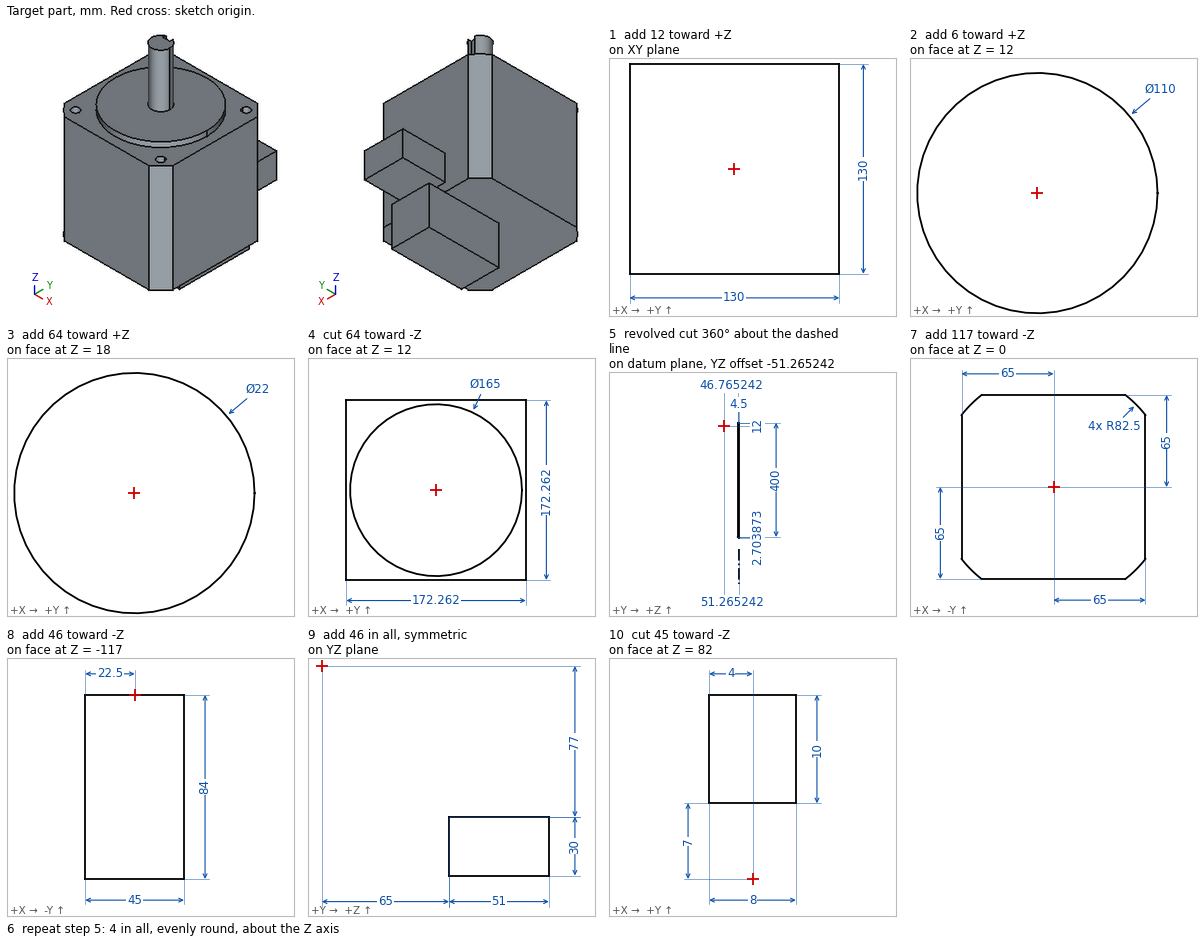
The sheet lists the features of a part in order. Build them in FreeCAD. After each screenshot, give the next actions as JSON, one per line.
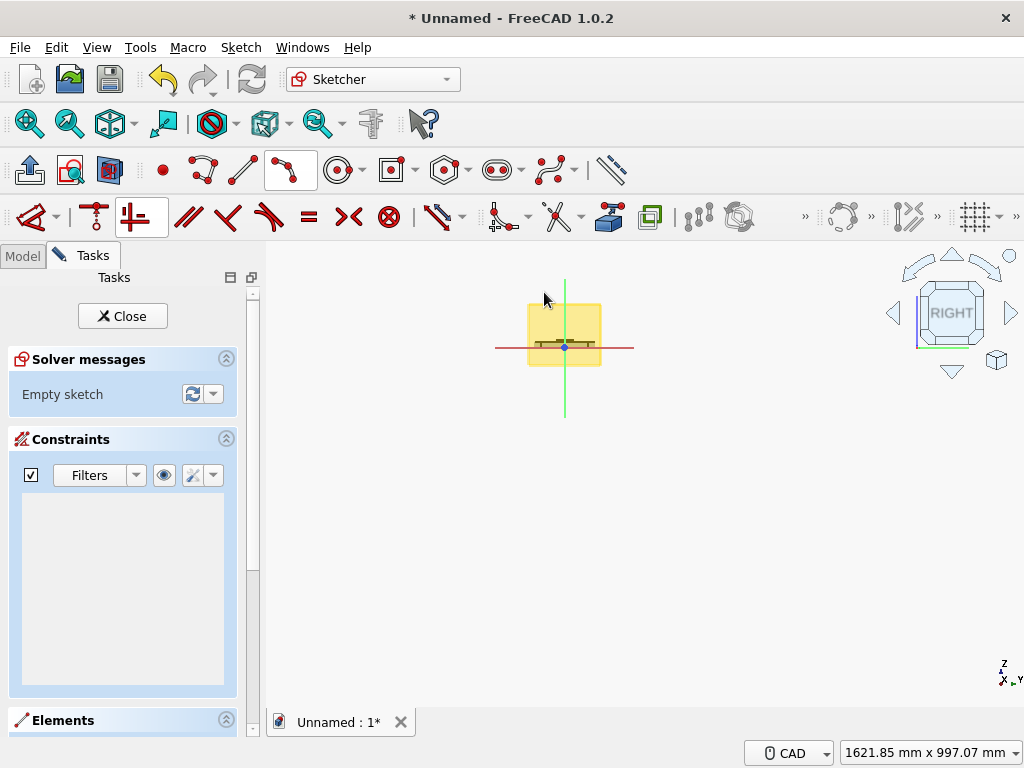
{"action": "left_click", "coordinate": [204, 170]}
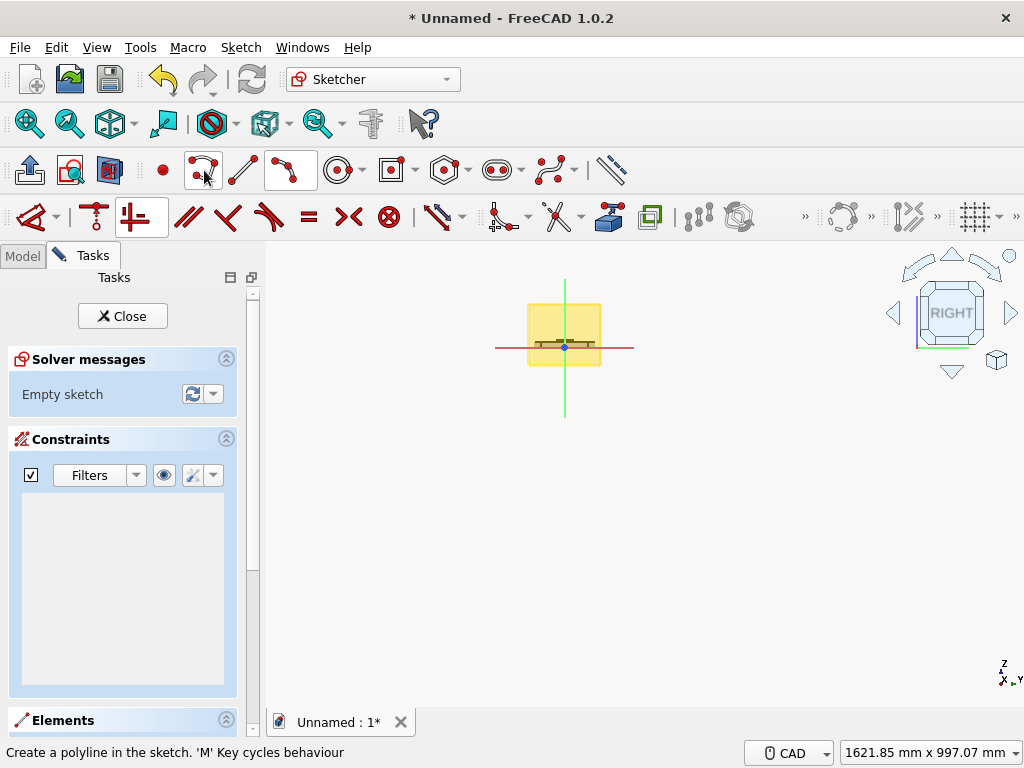
{"action": "scroll", "coordinate": [587, 342], "scroll_direction": "up", "scroll_amount": 6}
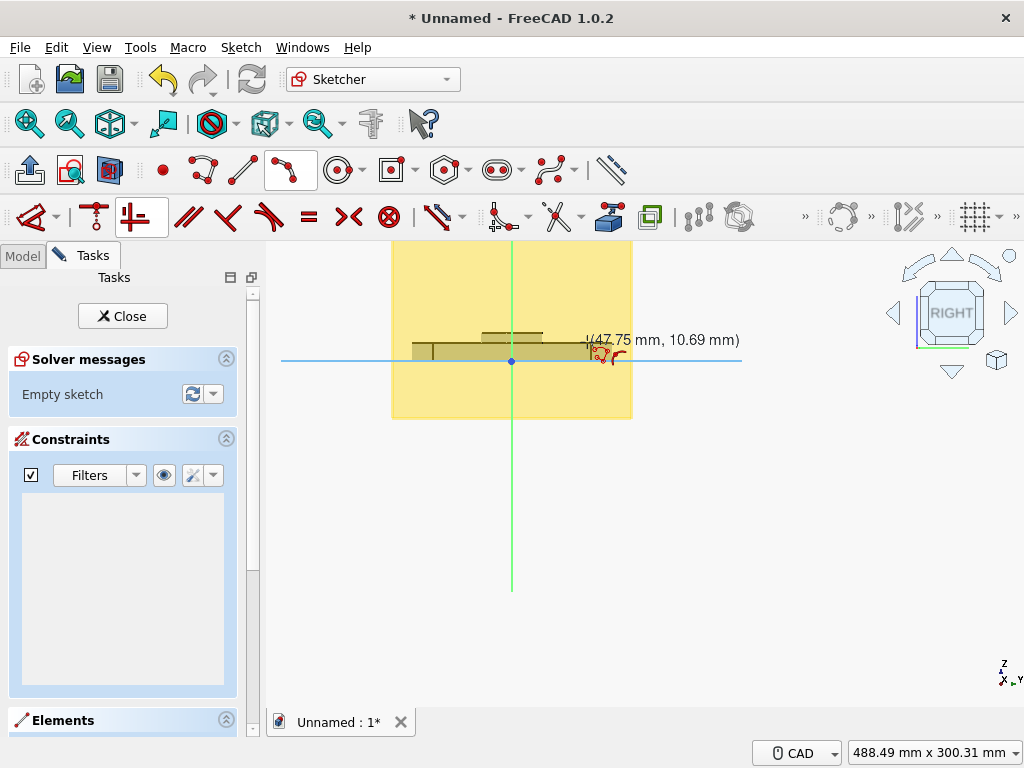
{"action": "left_click", "coordinate": [584, 343]}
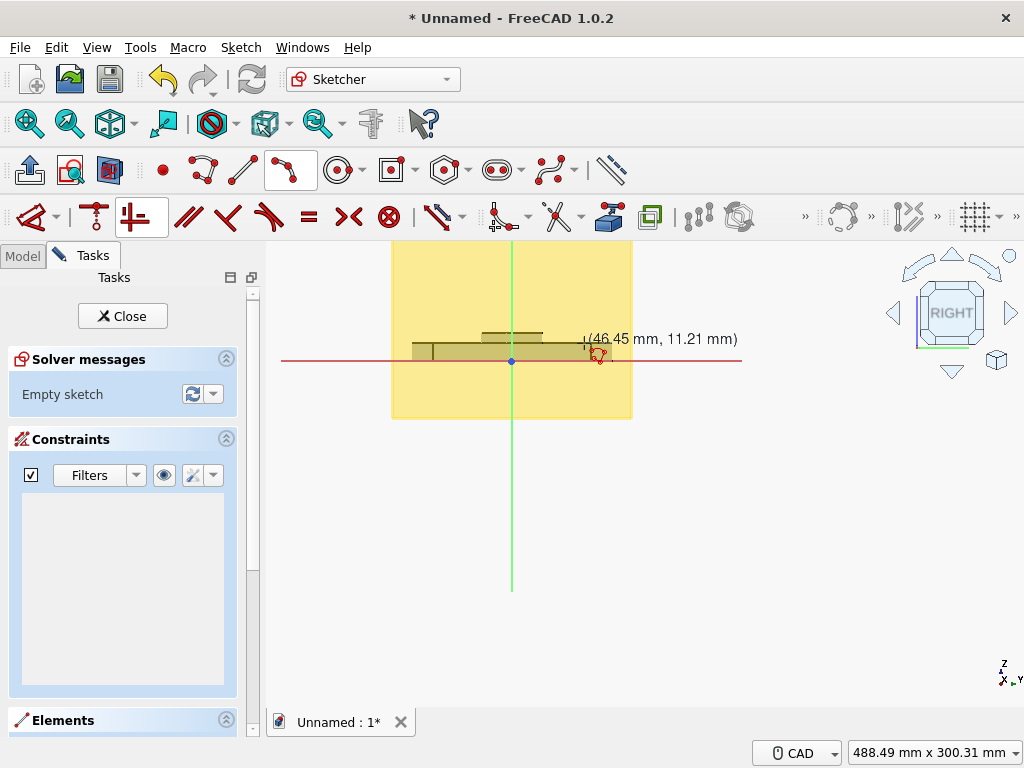
{"action": "scroll", "coordinate": [587, 342], "scroll_direction": "down", "scroll_amount": 6}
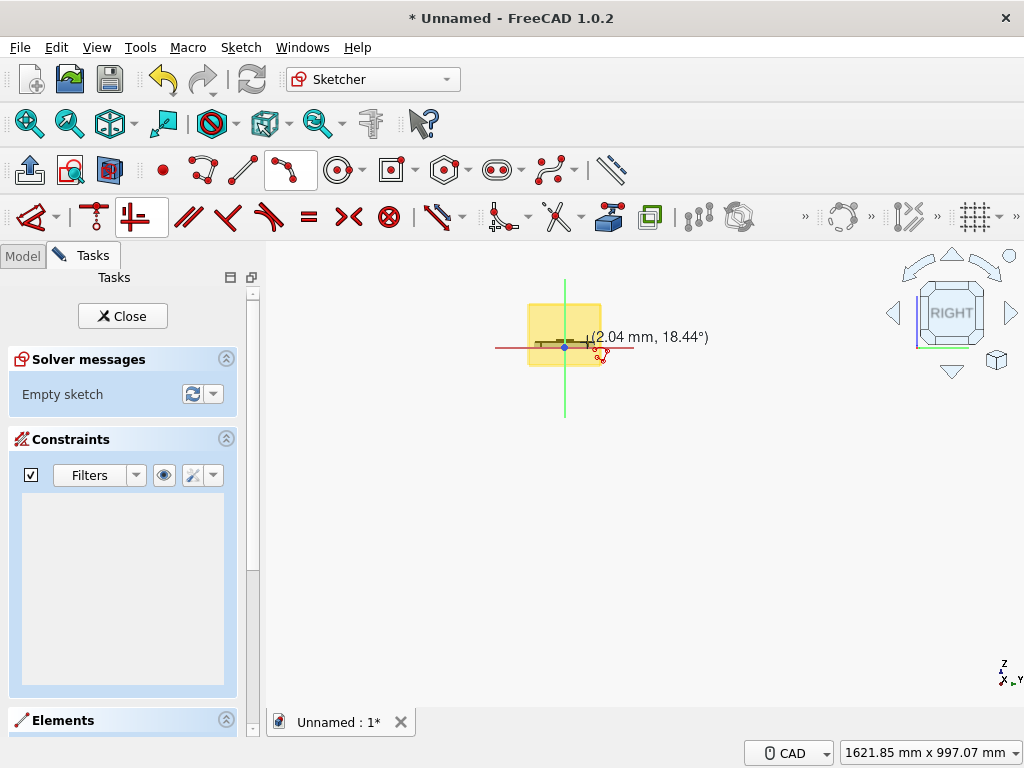
{"action": "left_click", "coordinate": [586, 529]}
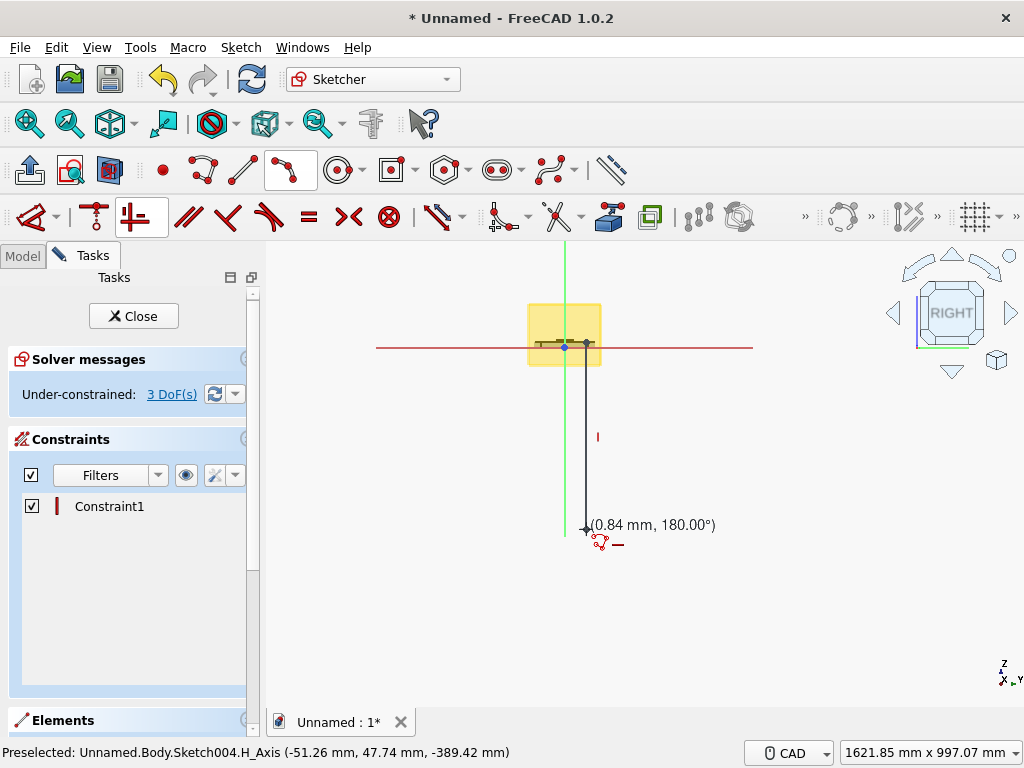
{"action": "scroll", "coordinate": [589, 531], "scroll_direction": "up", "scroll_amount": 10}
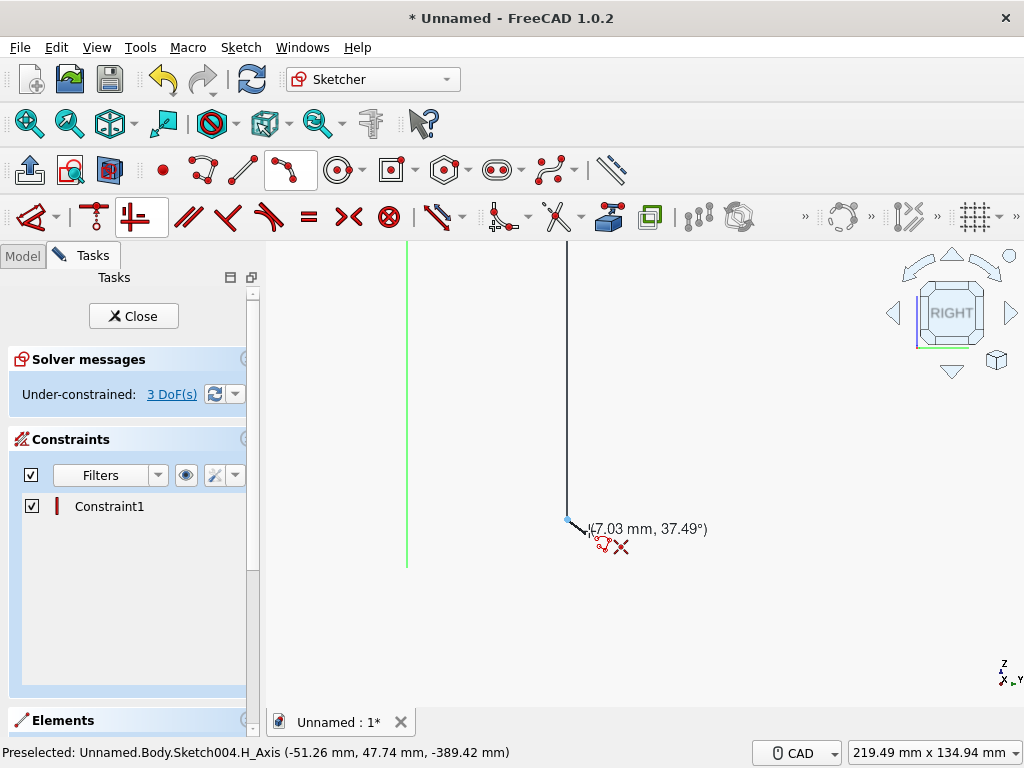
{"action": "left_click", "coordinate": [584, 524]}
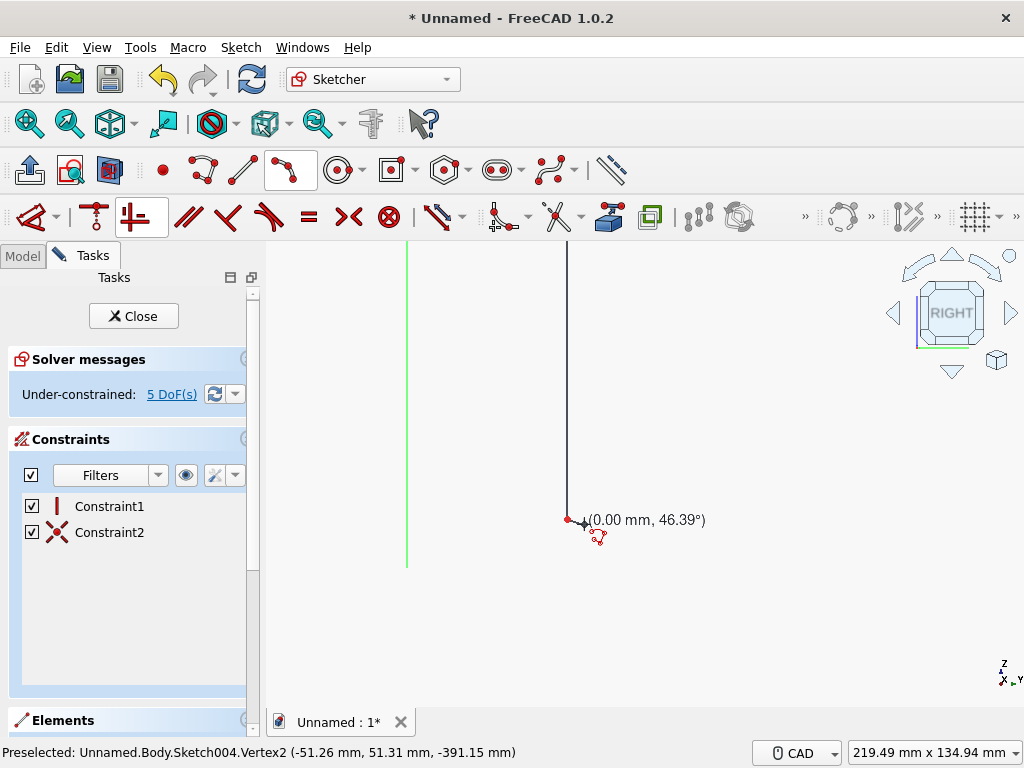
{"action": "scroll", "coordinate": [589, 531], "scroll_direction": "down", "scroll_amount": 10}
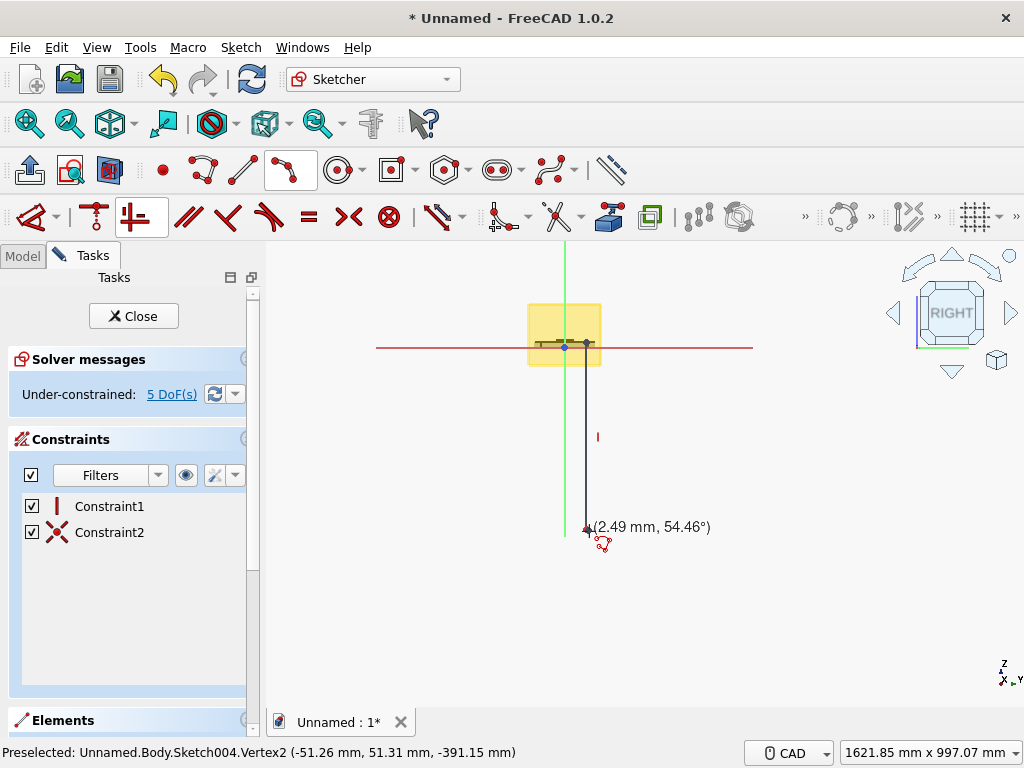
{"action": "scroll", "coordinate": [589, 342], "scroll_direction": "up", "scroll_amount": 11}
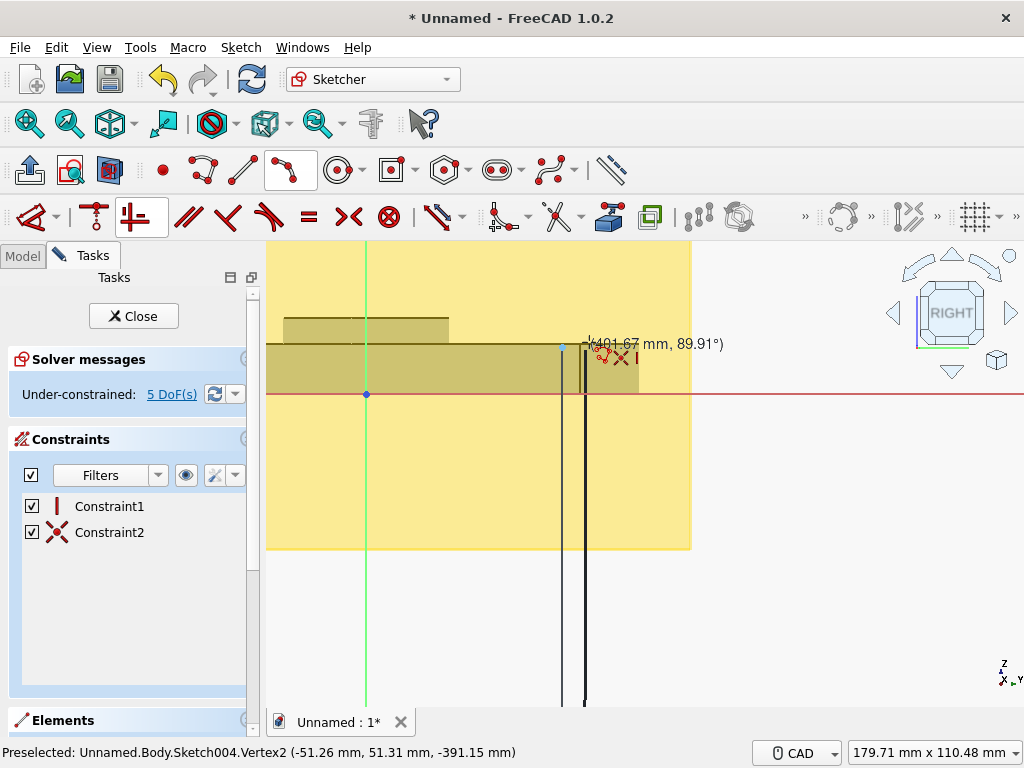
{"action": "left_click", "coordinate": [583, 344]}
{"action": "left_click", "coordinate": [562, 347]}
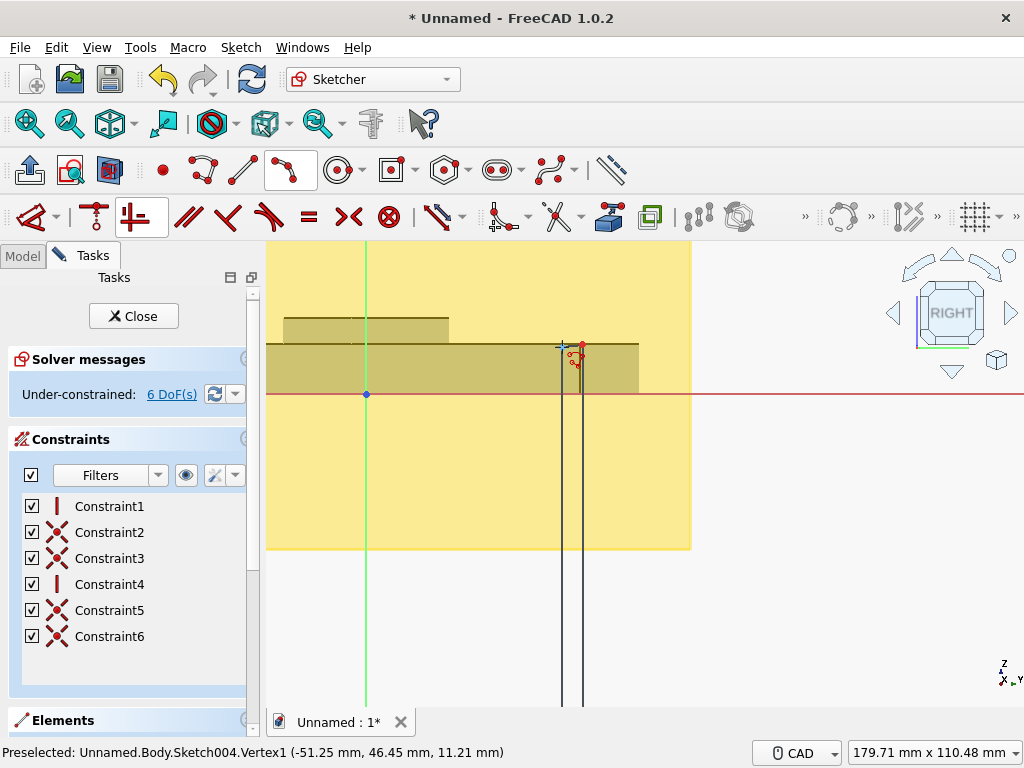
{"action": "left_click", "coordinate": [244, 170]}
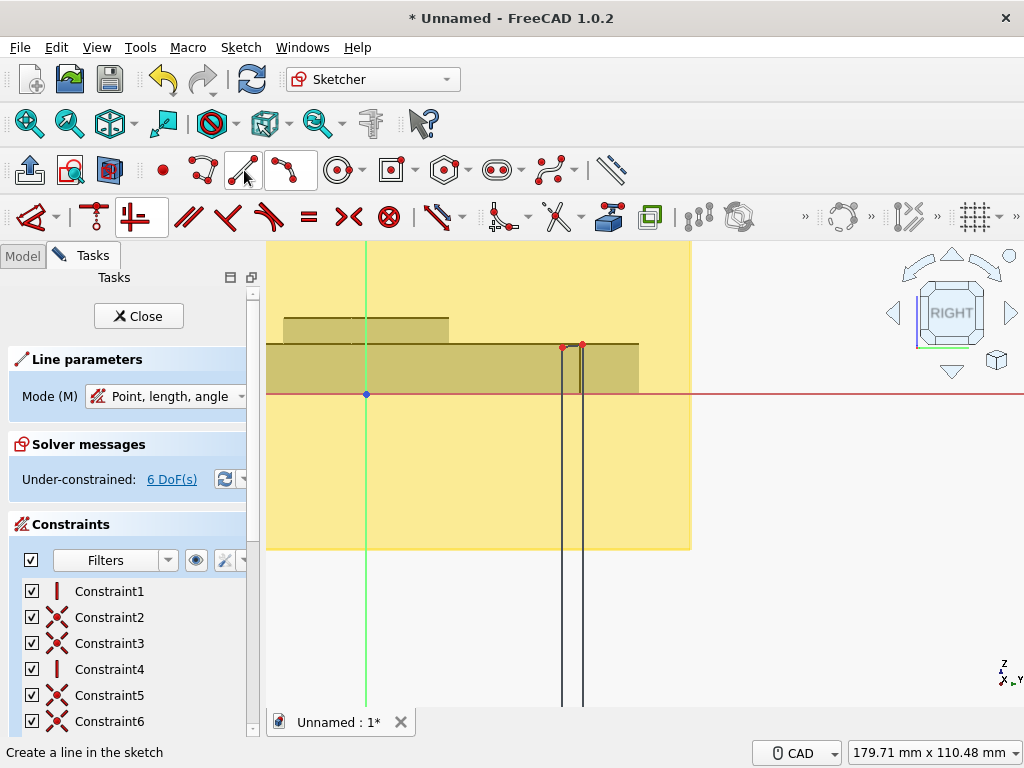
{"action": "scroll", "coordinate": [589, 342], "scroll_direction": "down", "scroll_amount": 11}